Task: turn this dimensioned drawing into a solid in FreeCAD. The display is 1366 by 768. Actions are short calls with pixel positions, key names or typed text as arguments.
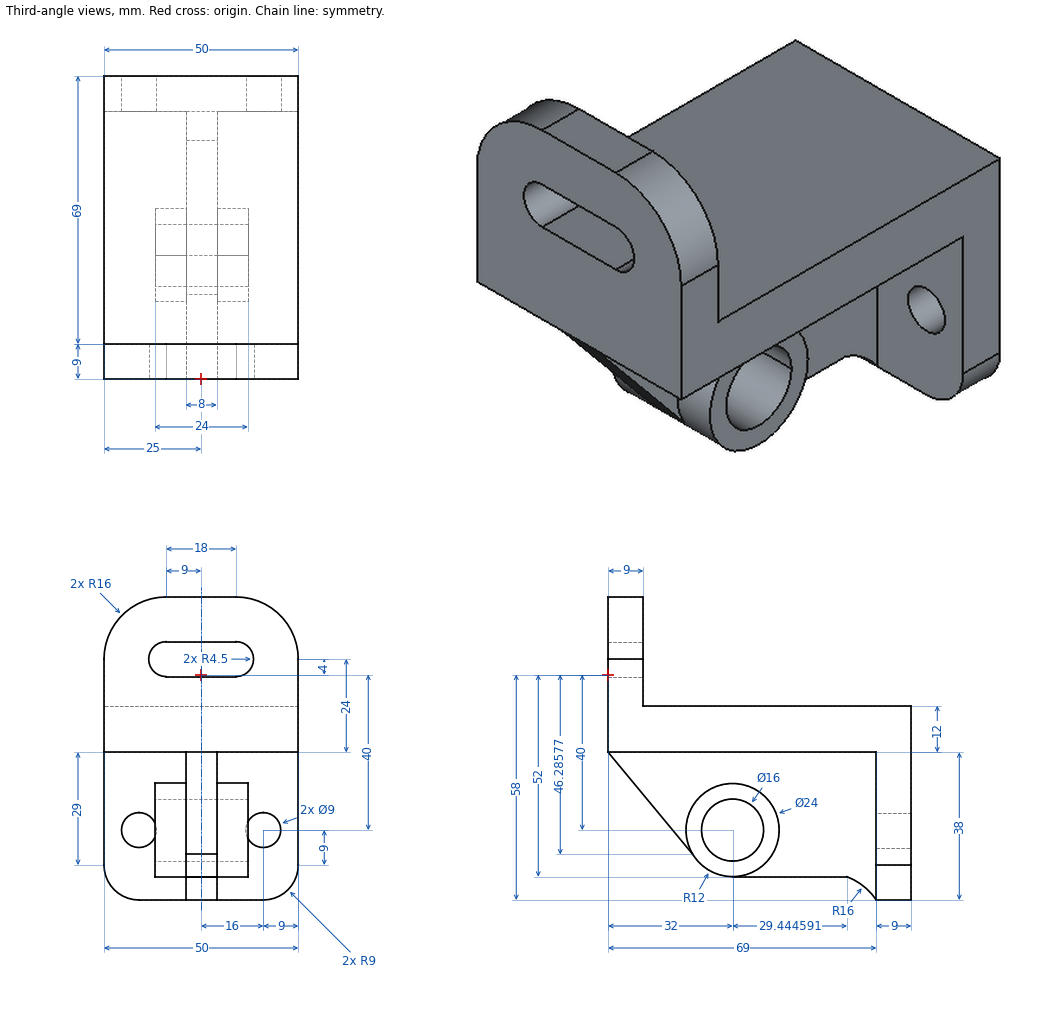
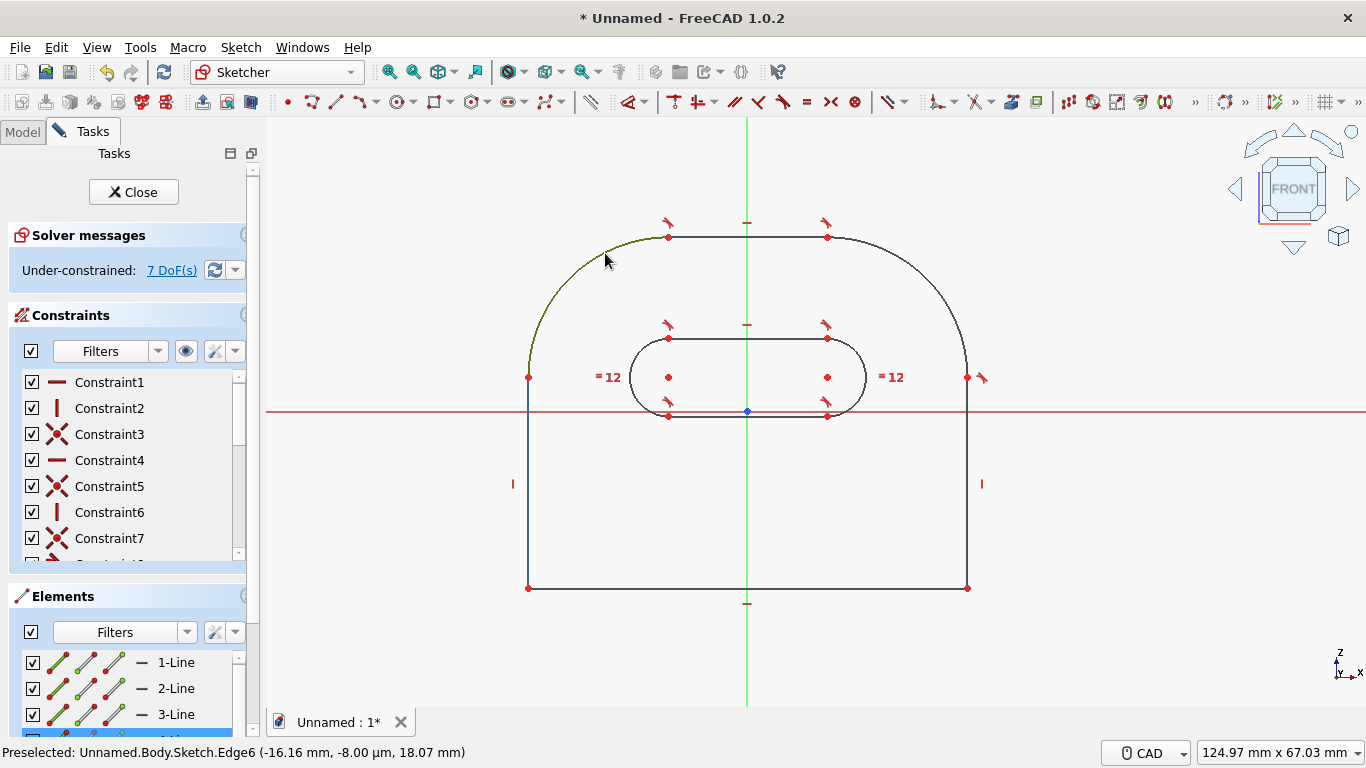
click(784, 102)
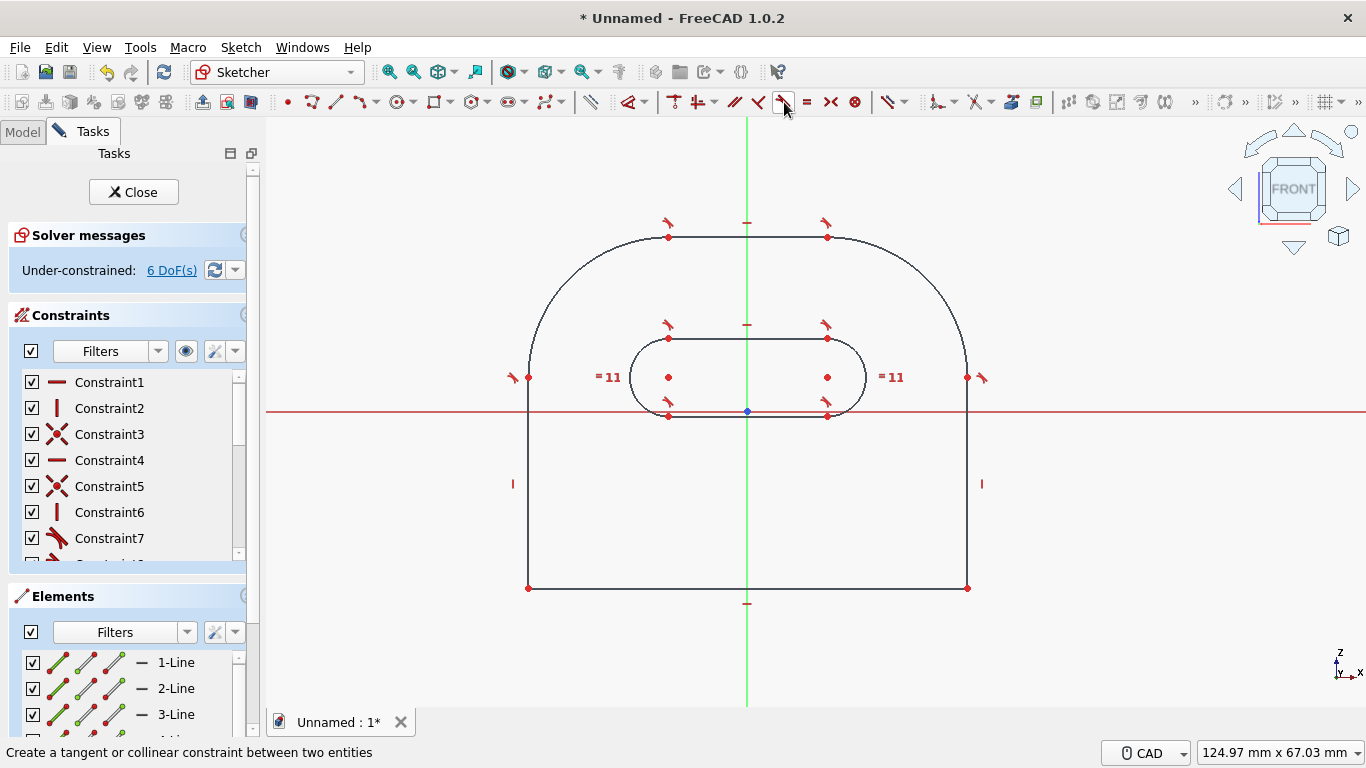
key(d)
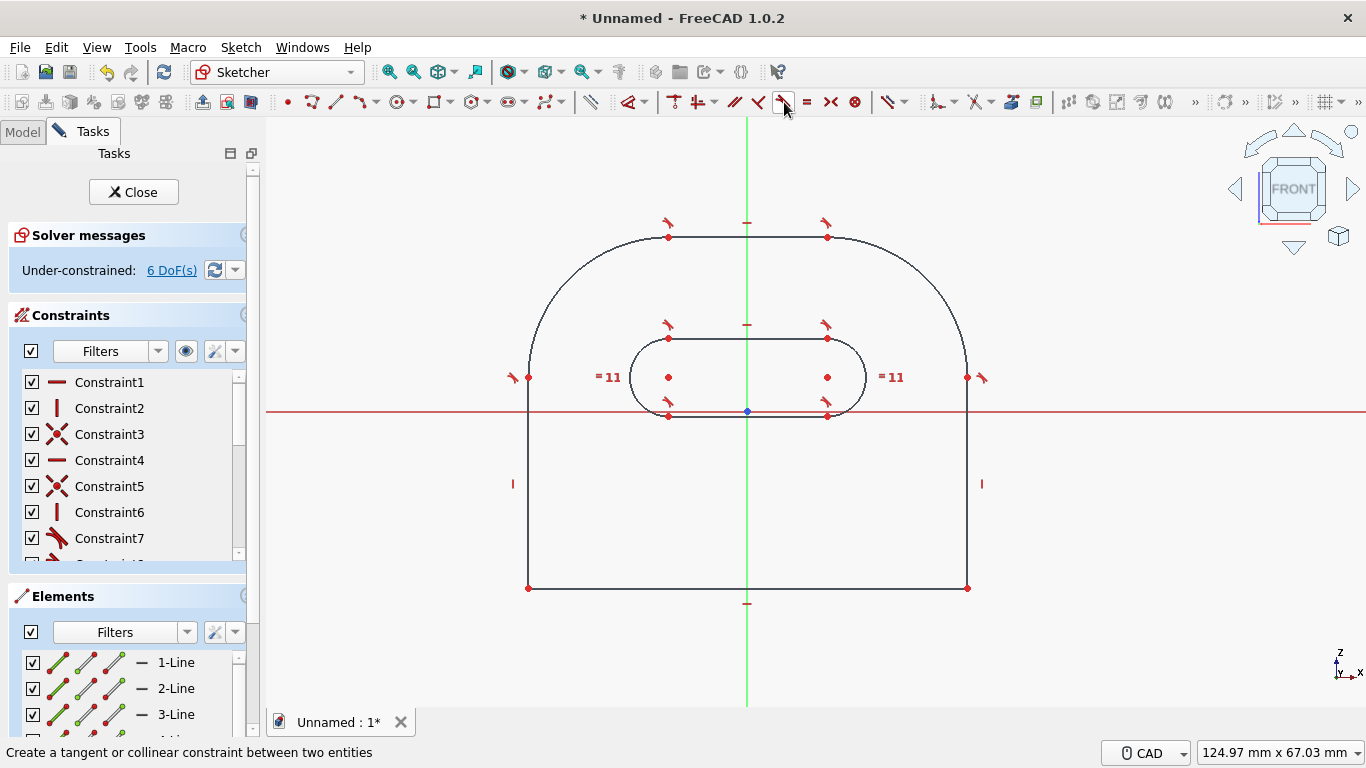
click(952, 314)
click(981, 299)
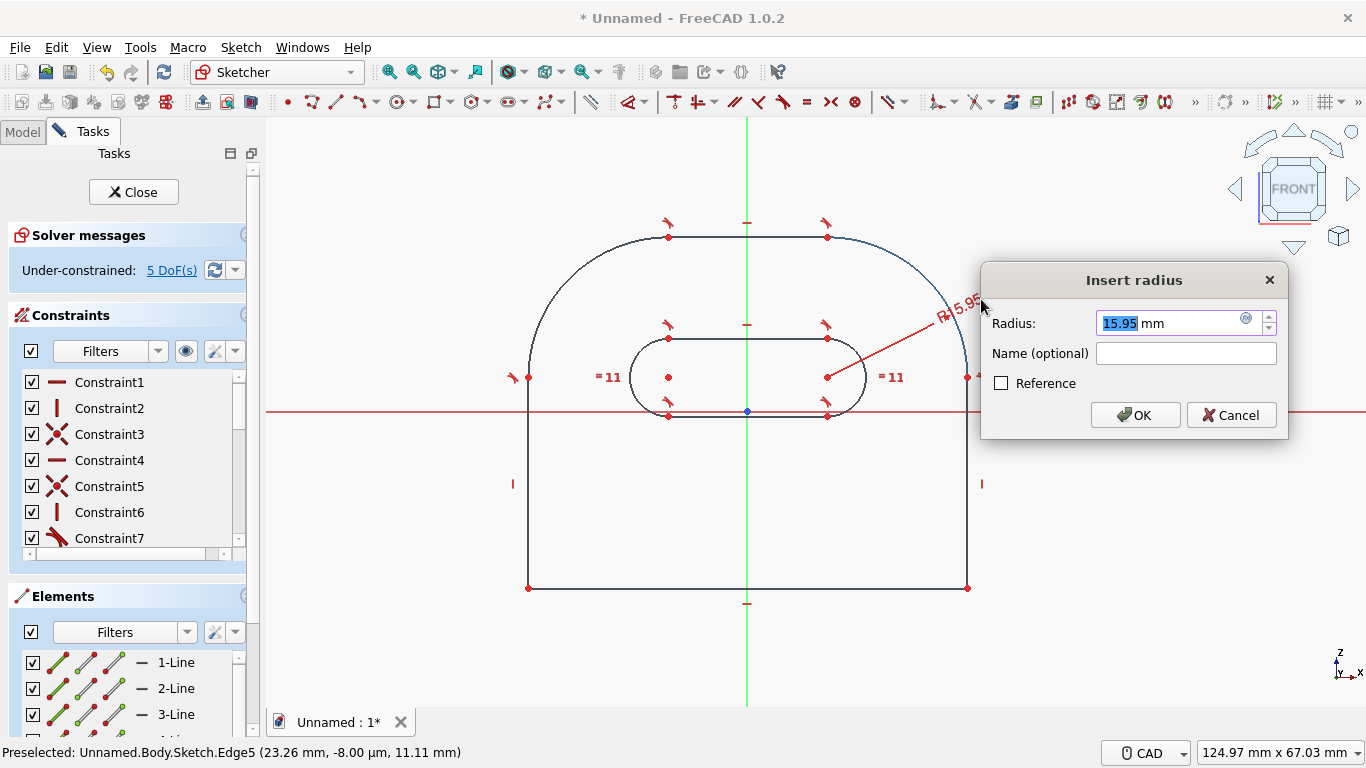
text(16)
key(Return)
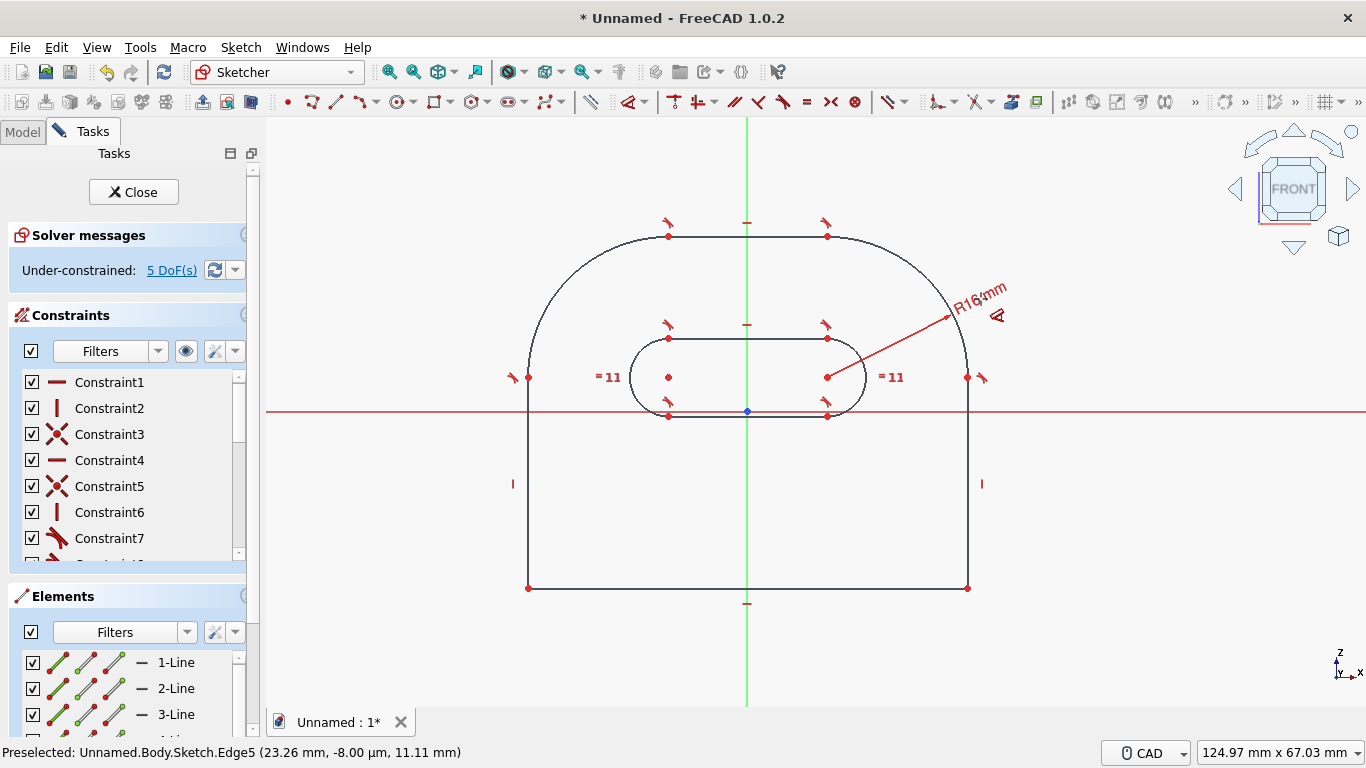
click(637, 355)
click(611, 336)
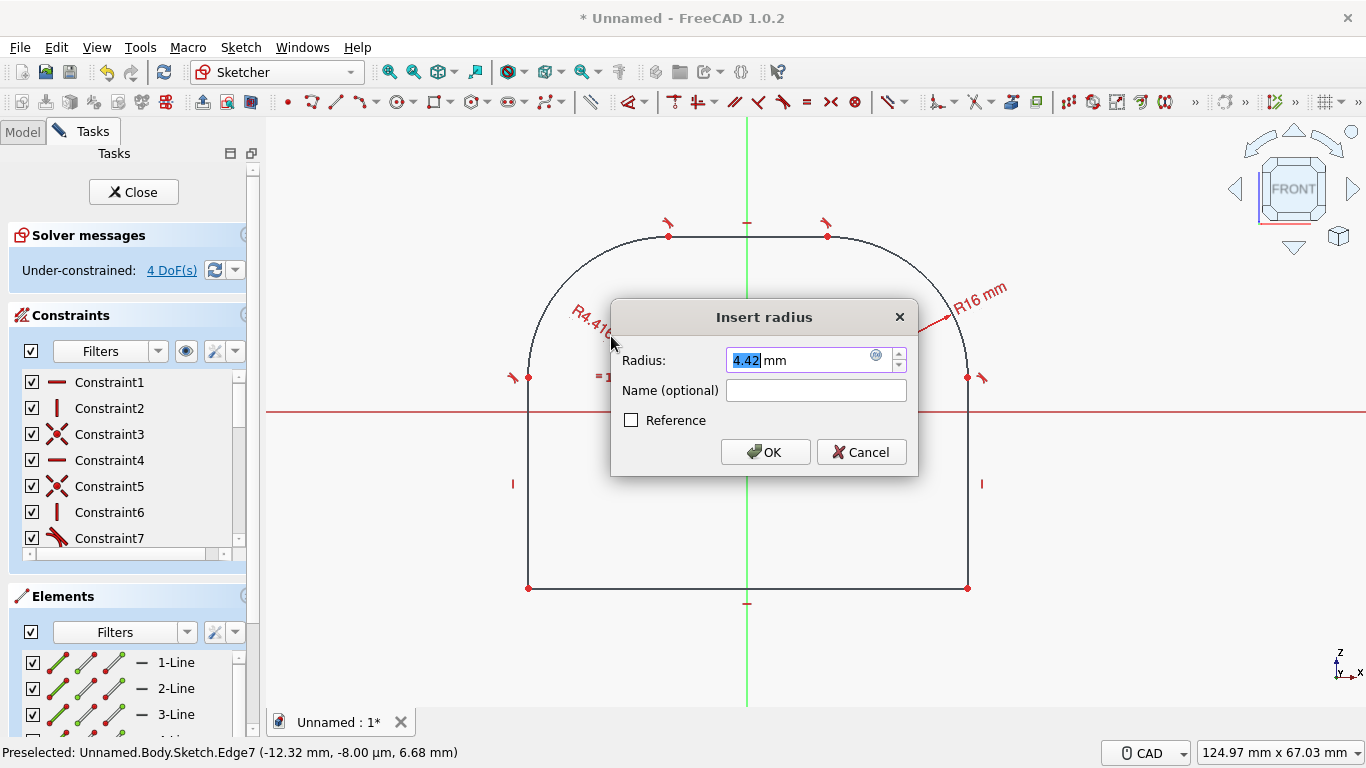
text(4.5)
key(Return)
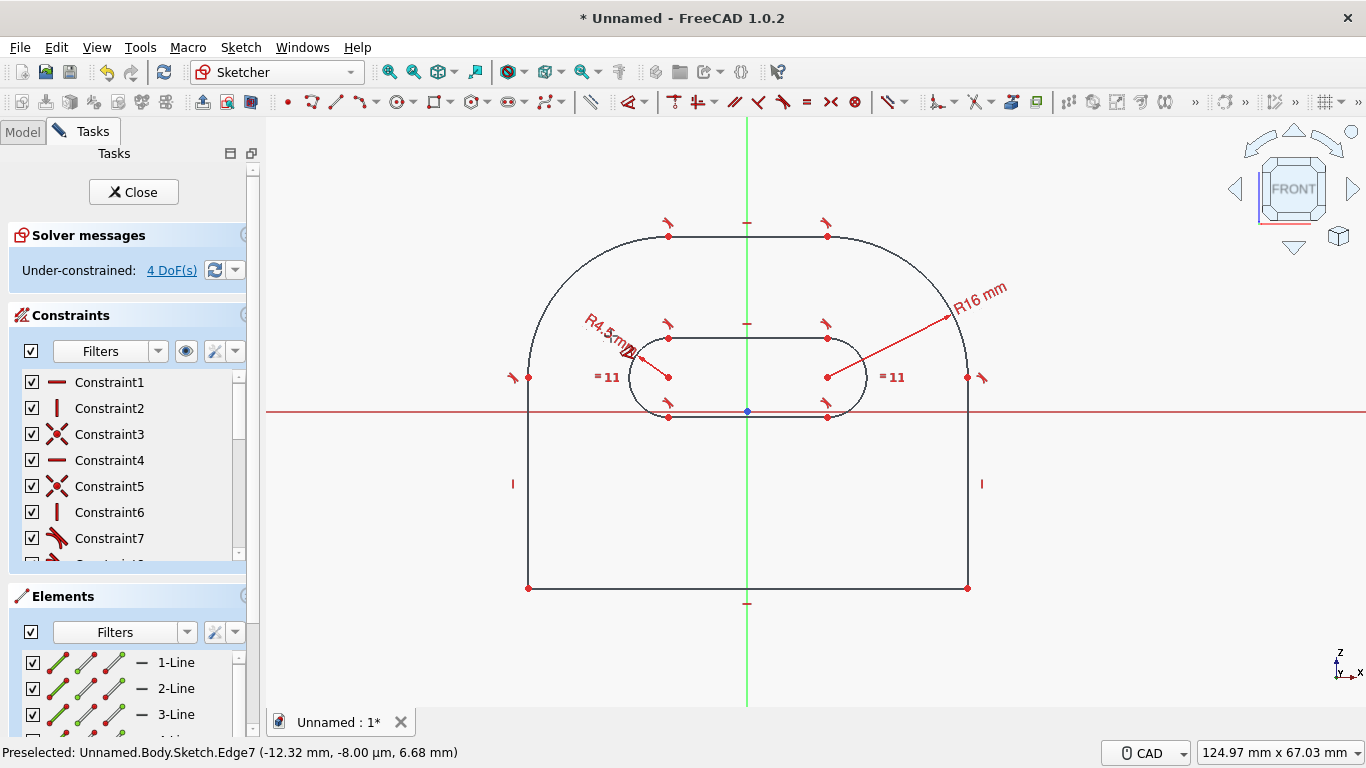
click(716, 237)
click(712, 203)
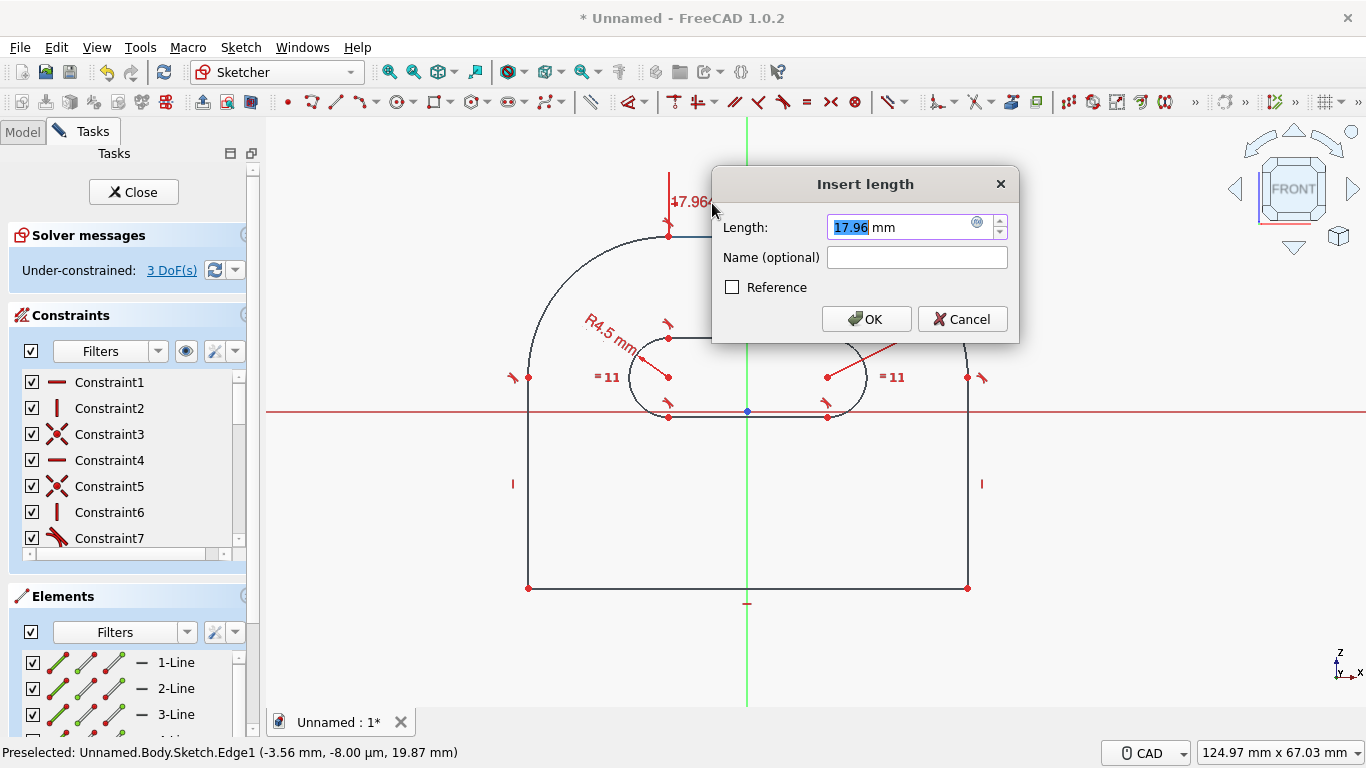
text(18)
key(Return)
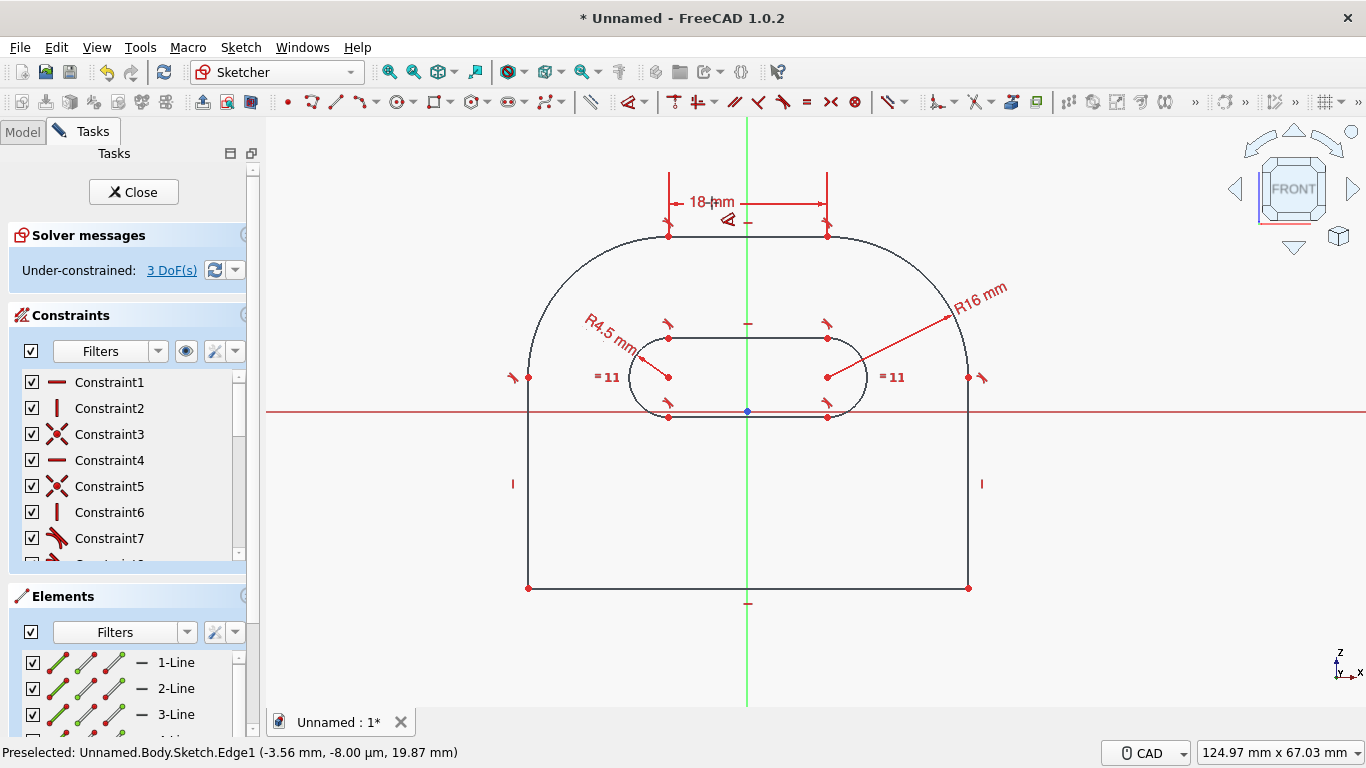
click(968, 441)
click(1002, 483)